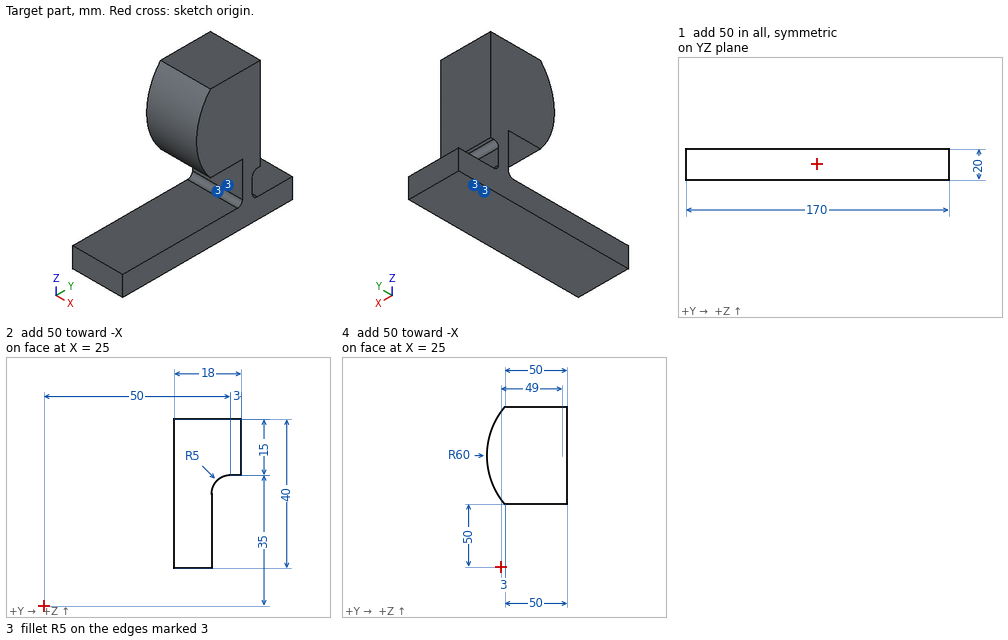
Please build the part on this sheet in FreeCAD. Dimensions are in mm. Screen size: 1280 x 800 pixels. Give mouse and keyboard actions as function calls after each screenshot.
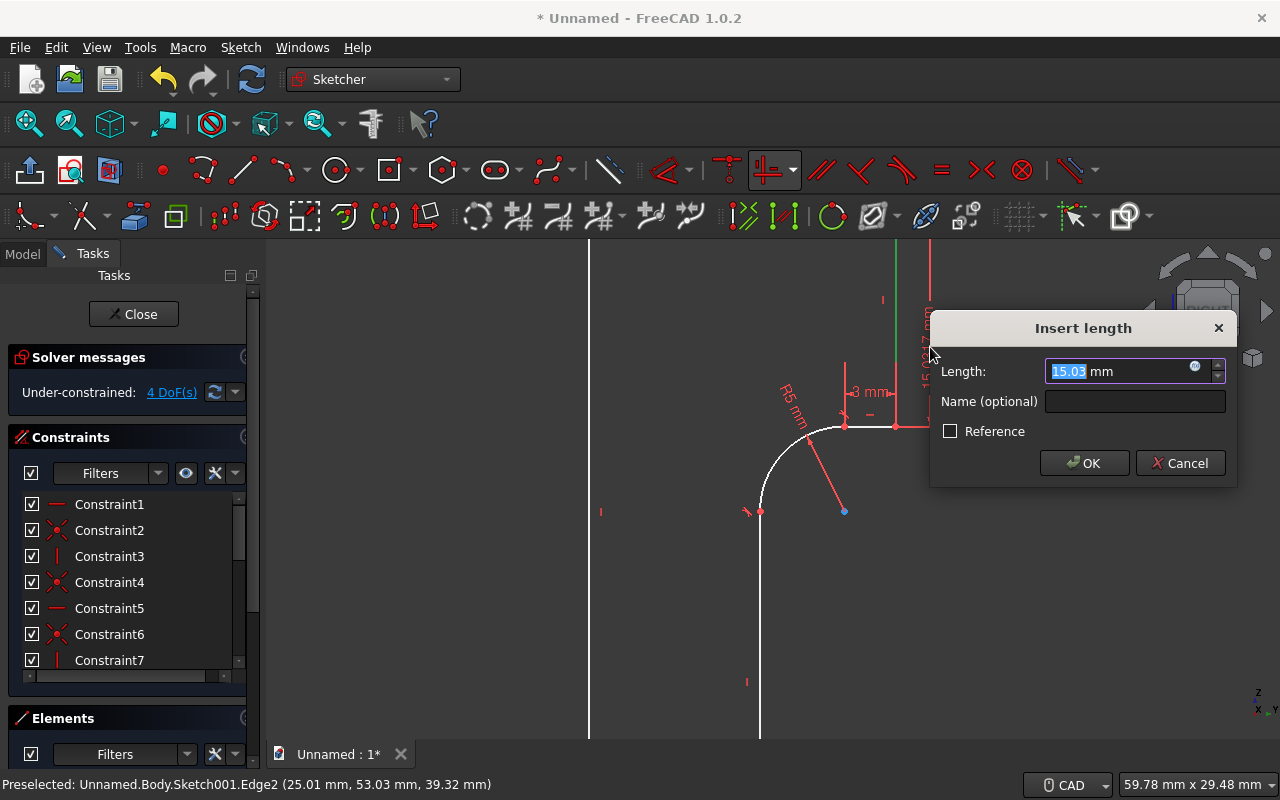
text(15)
key(Return)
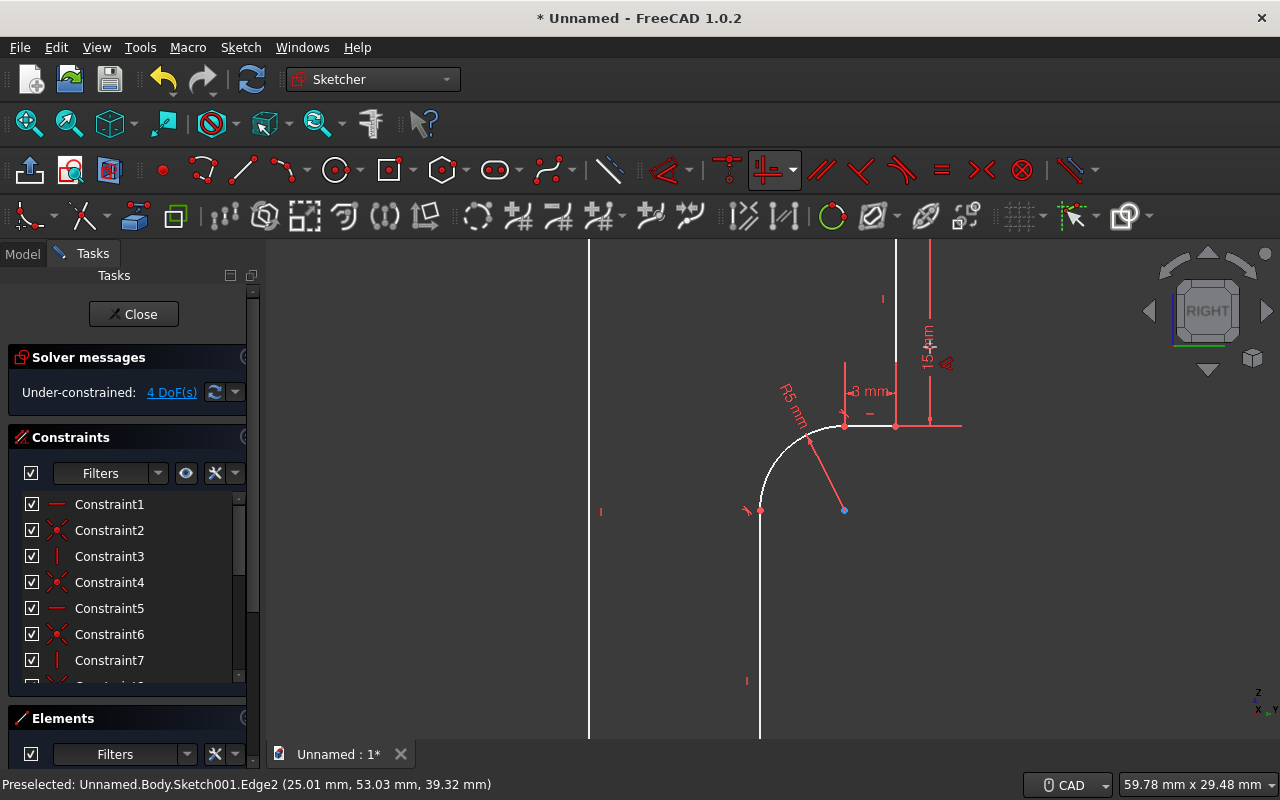
scroll(855, 428, down, 5)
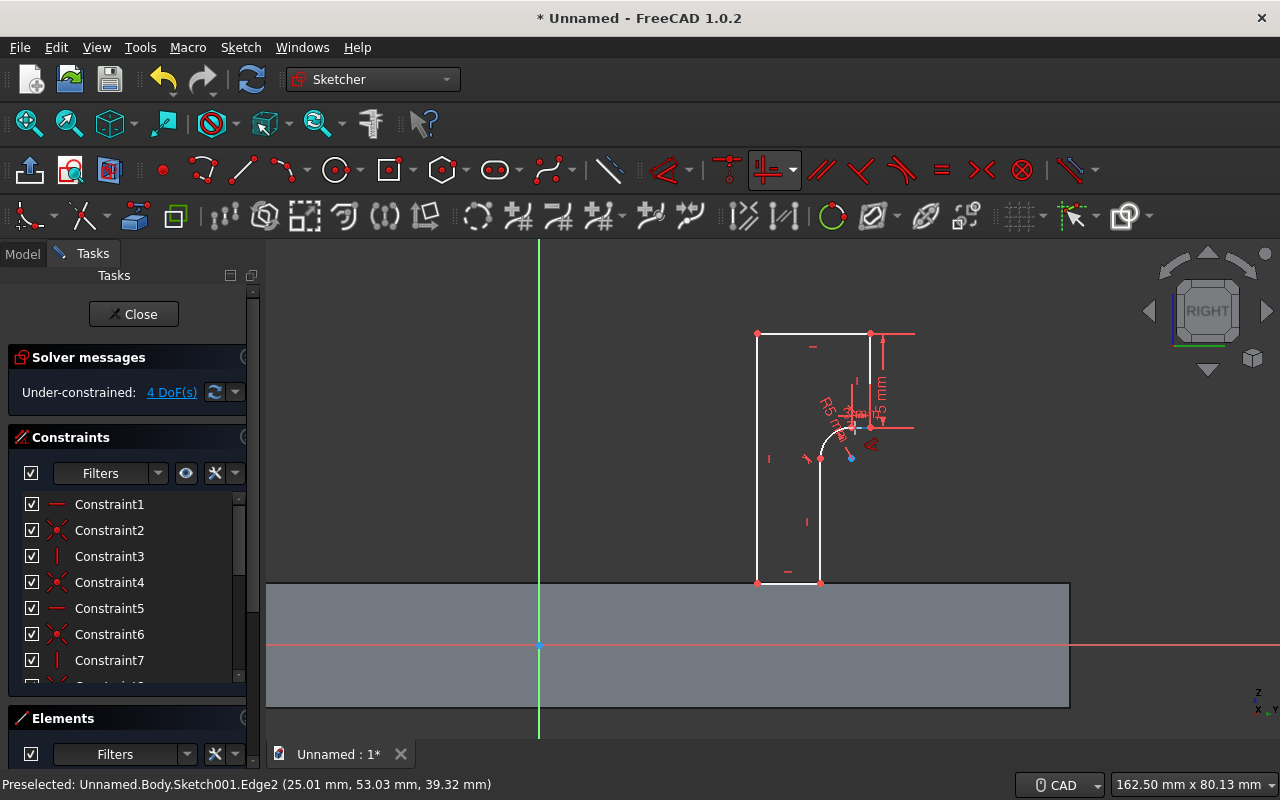
click(836, 334)
click(814, 300)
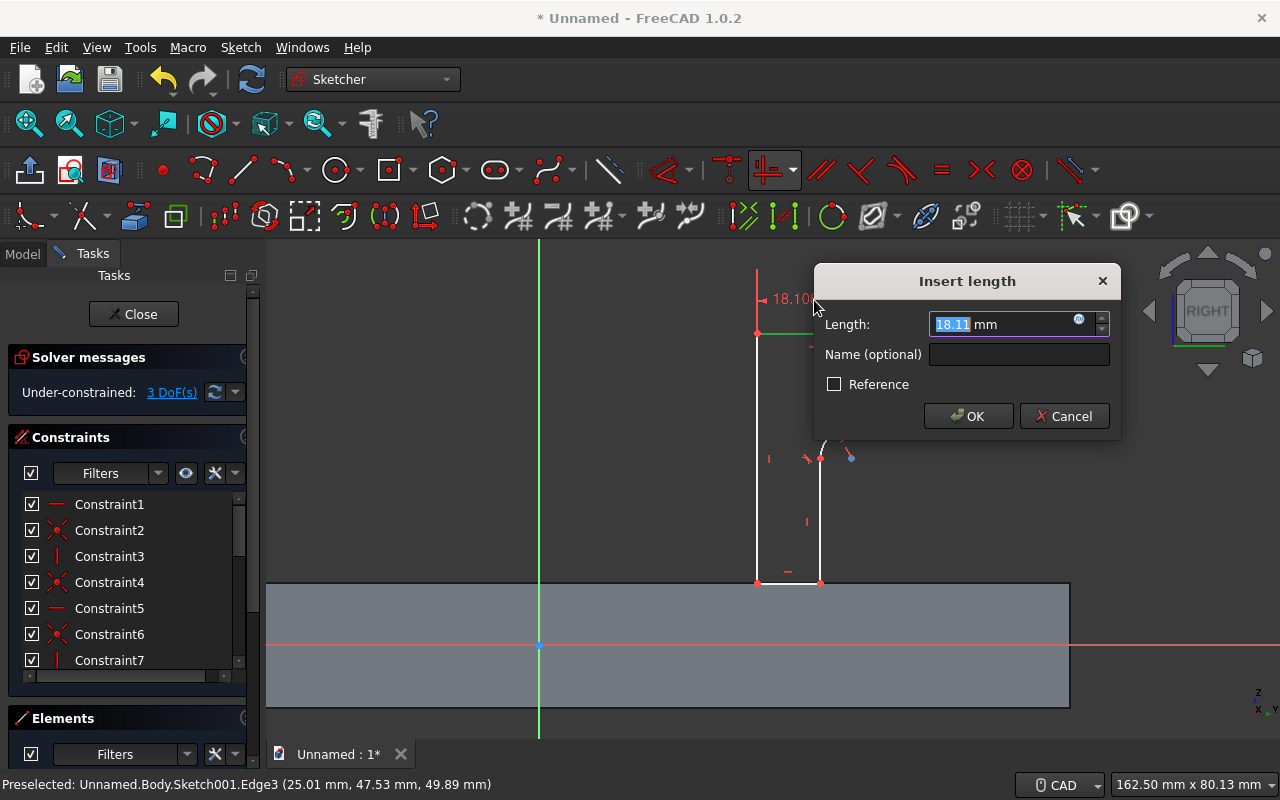
text(18)
key(Return)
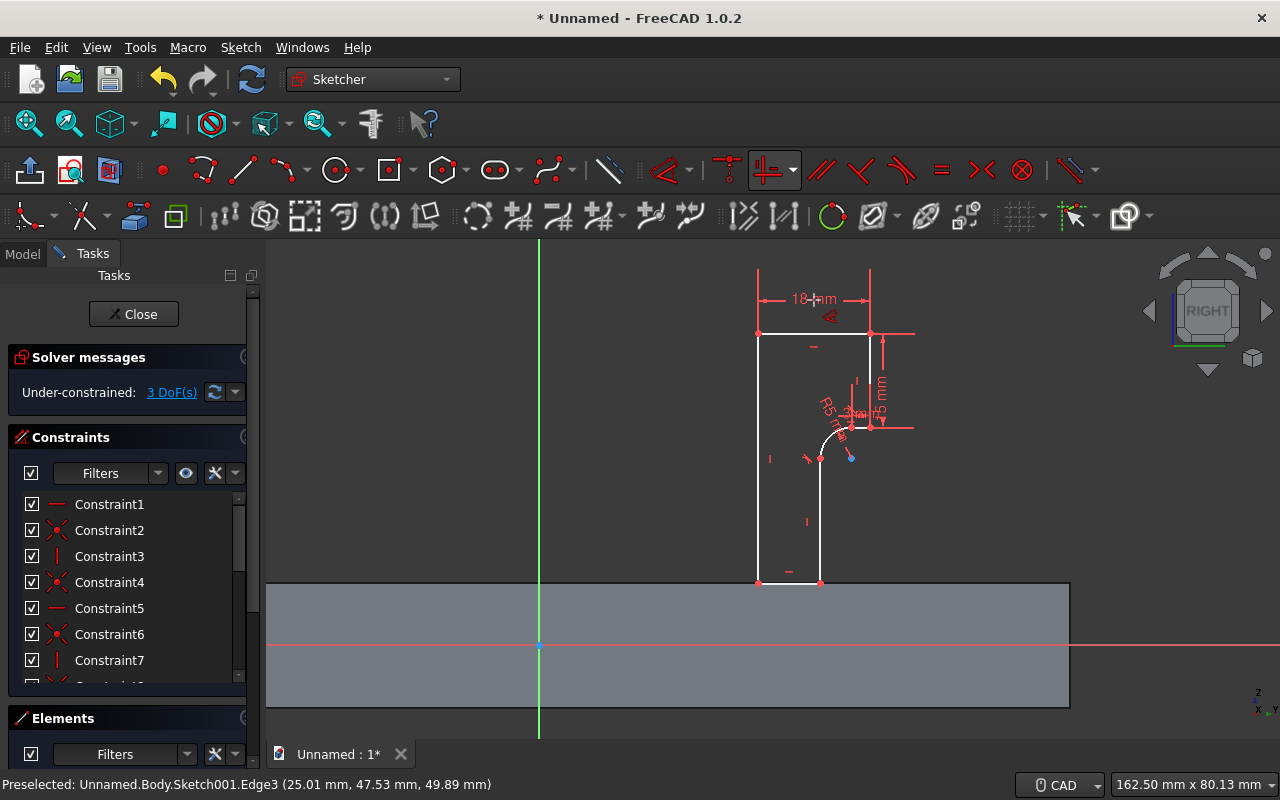
click(758, 409)
click(792, 459)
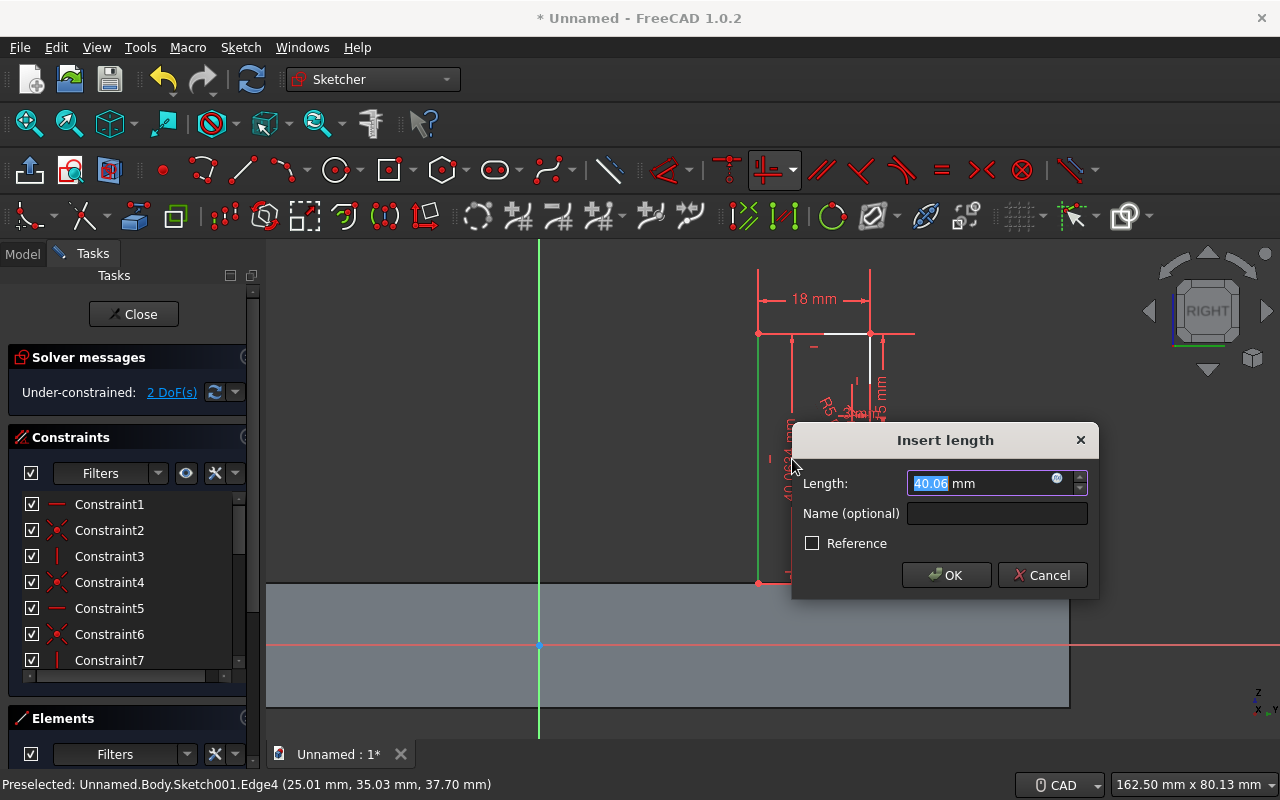
text(40)
key(Return)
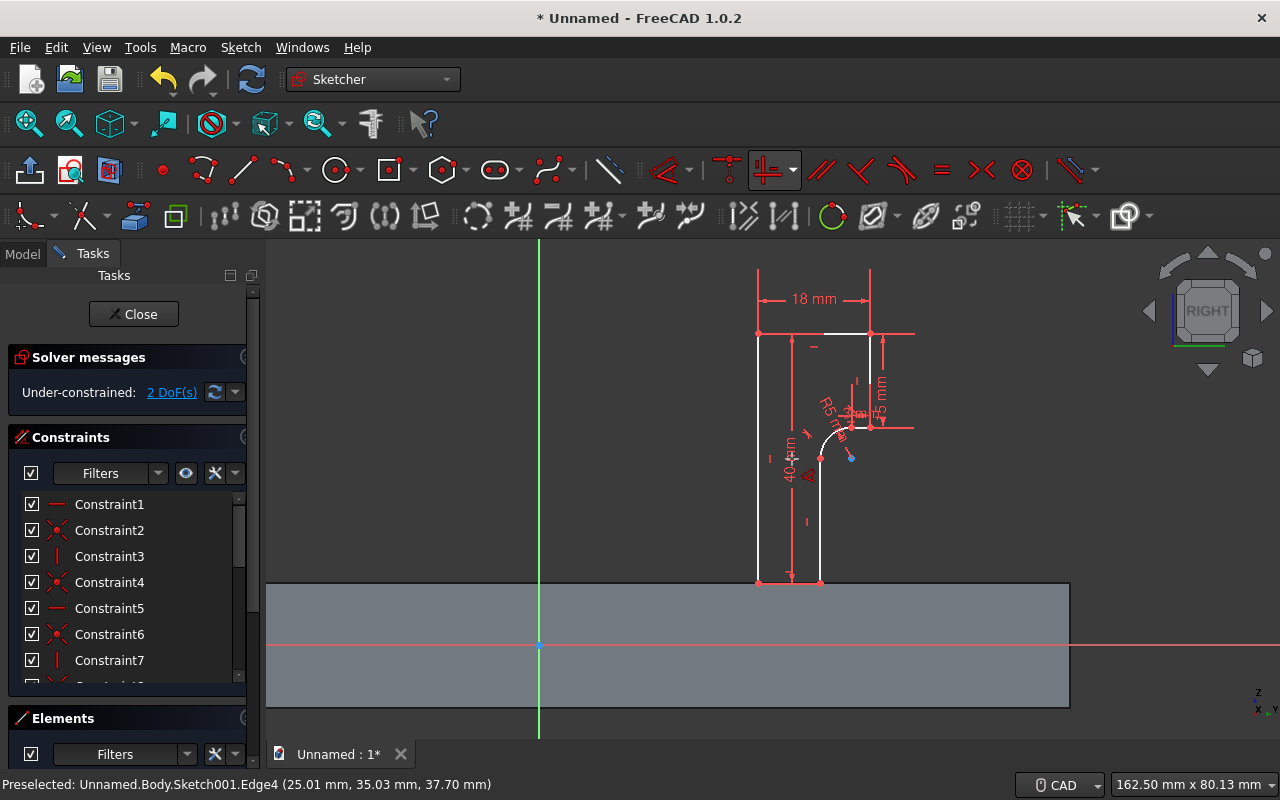
click(852, 428)
click(696, 679)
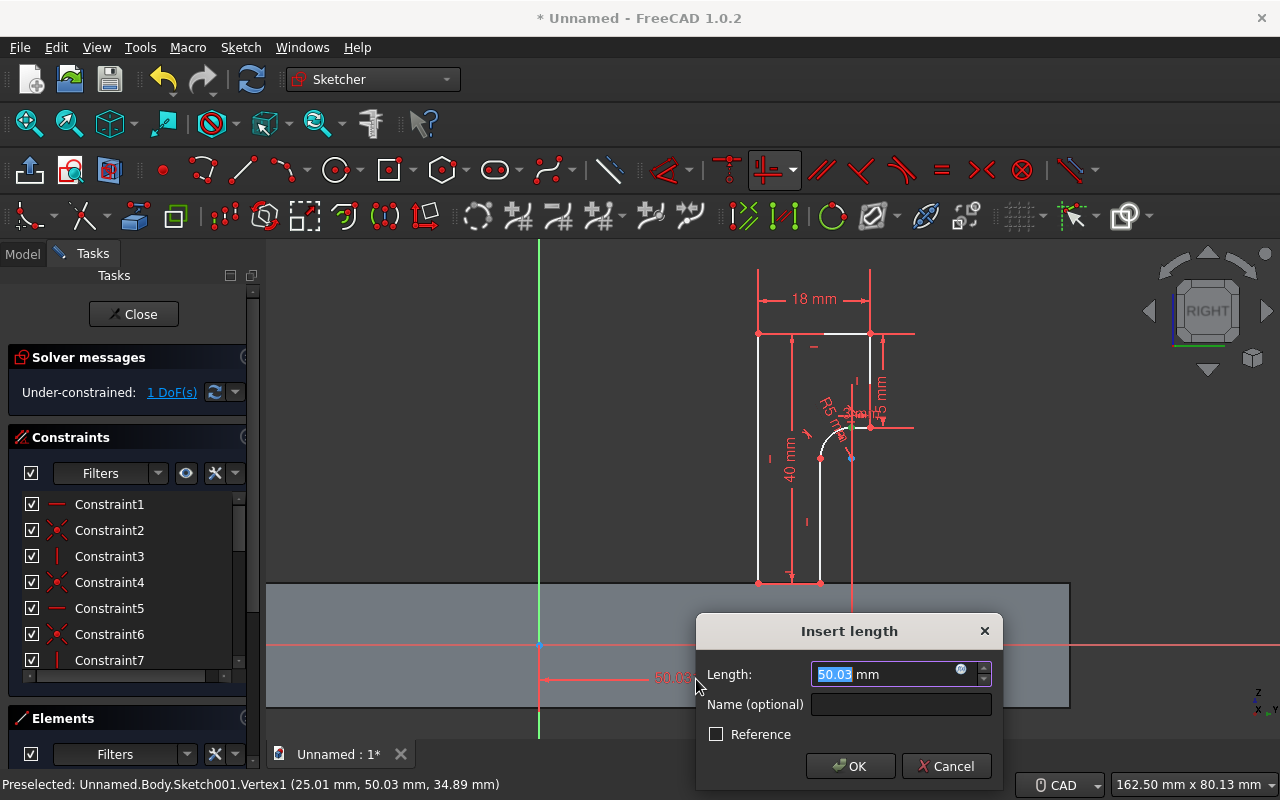
text(50)
key(Return)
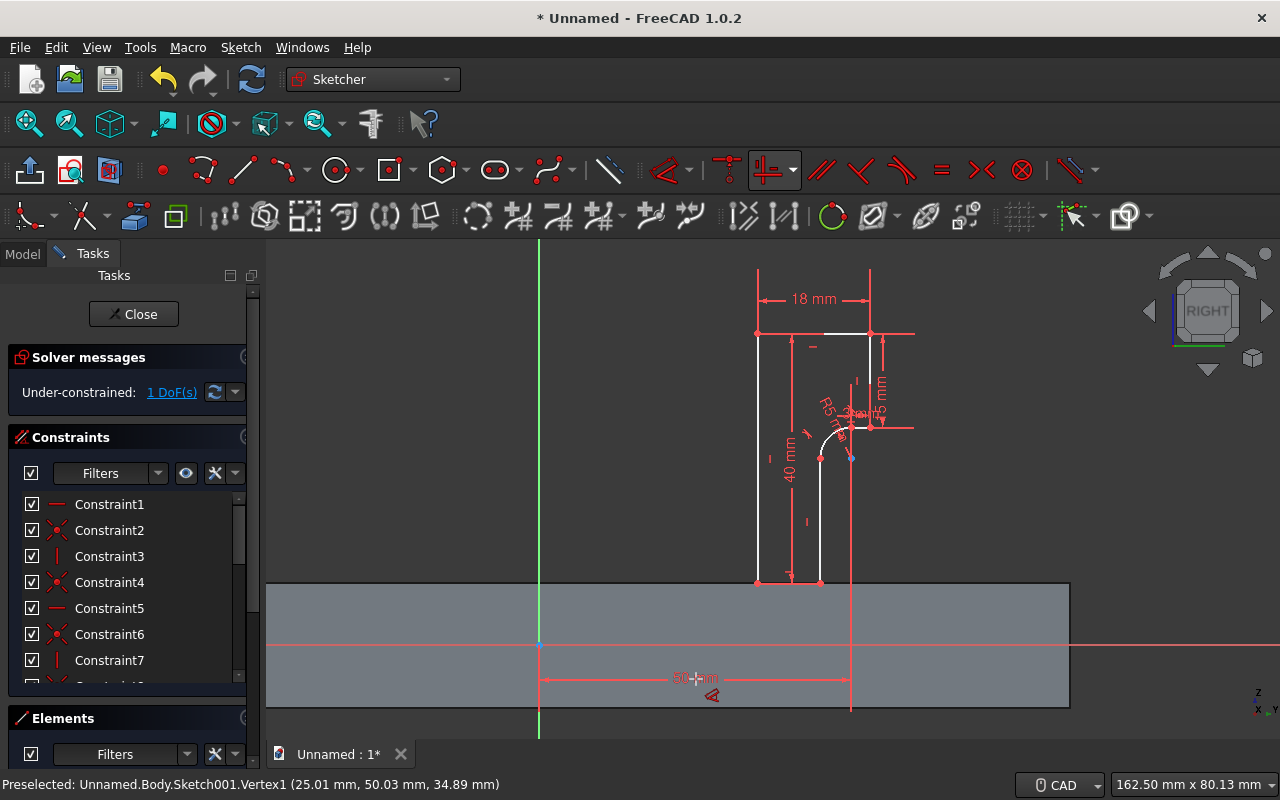
click(851, 428)
click(505, 536)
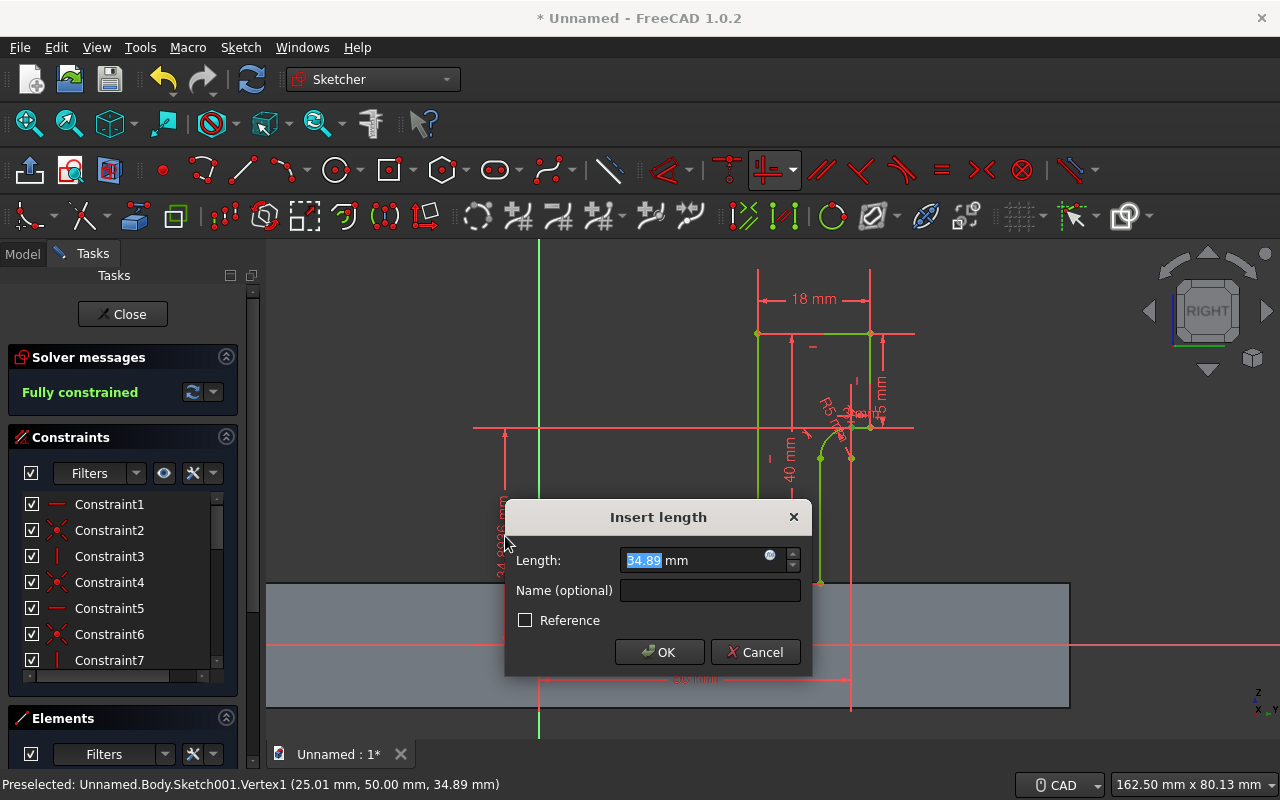
text(35)
key(Return)
key(Escape)